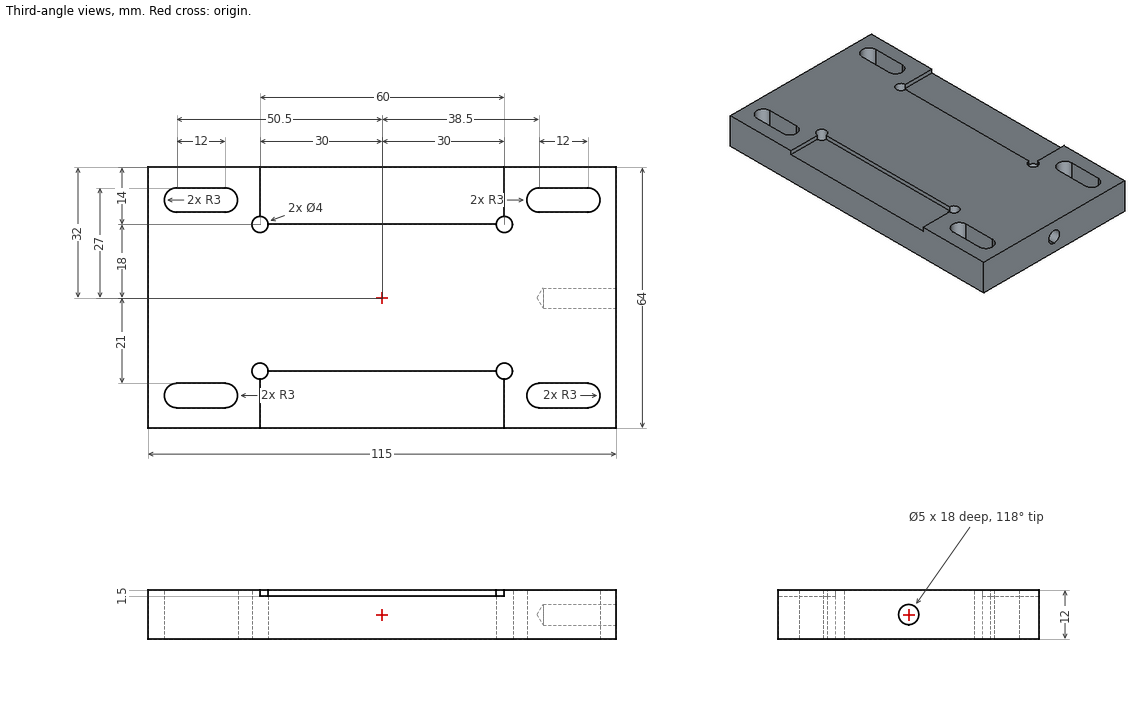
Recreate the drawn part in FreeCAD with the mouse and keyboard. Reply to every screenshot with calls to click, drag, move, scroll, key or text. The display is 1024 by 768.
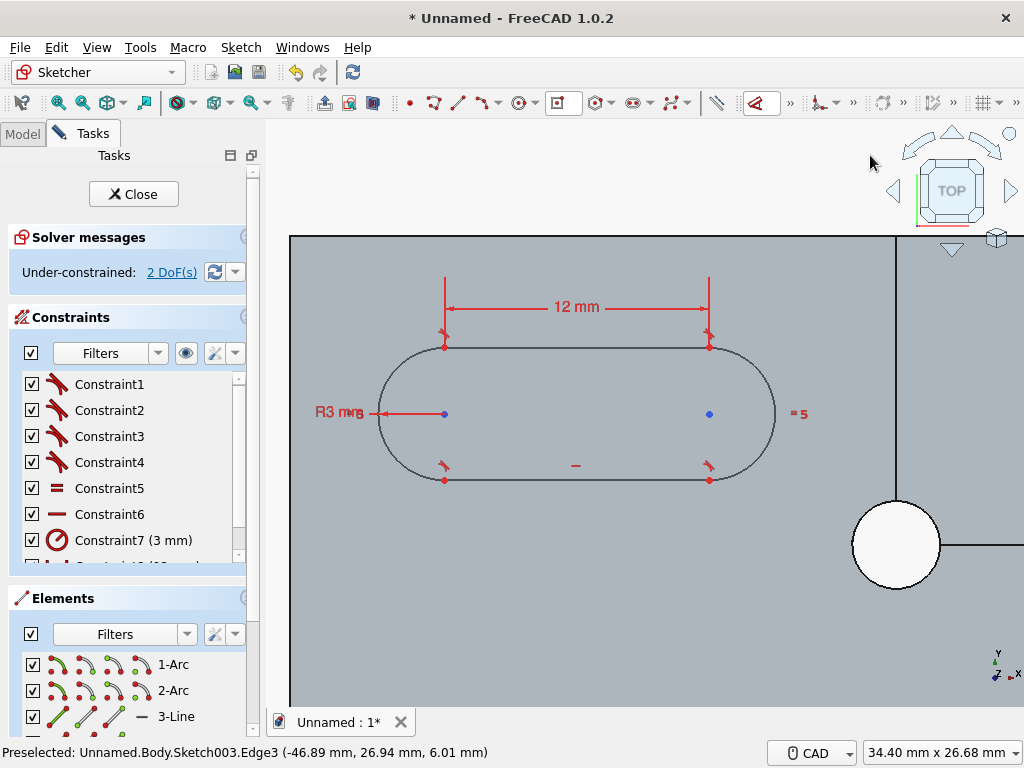
click(445, 348)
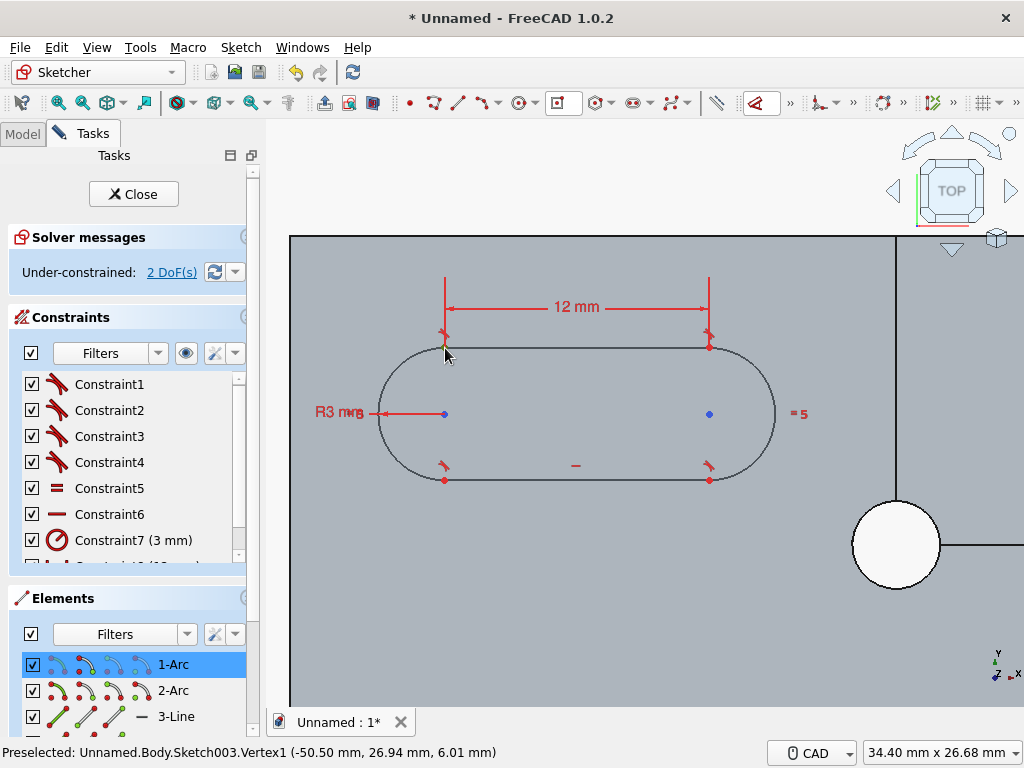
key(i)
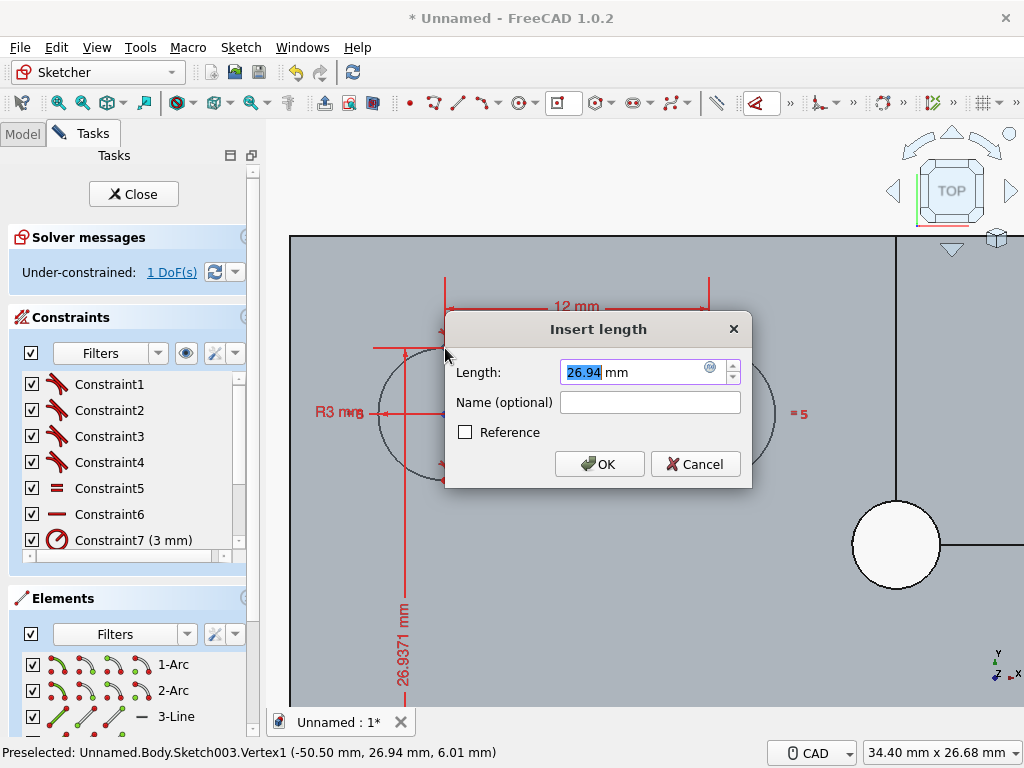
text(27)
key(Return)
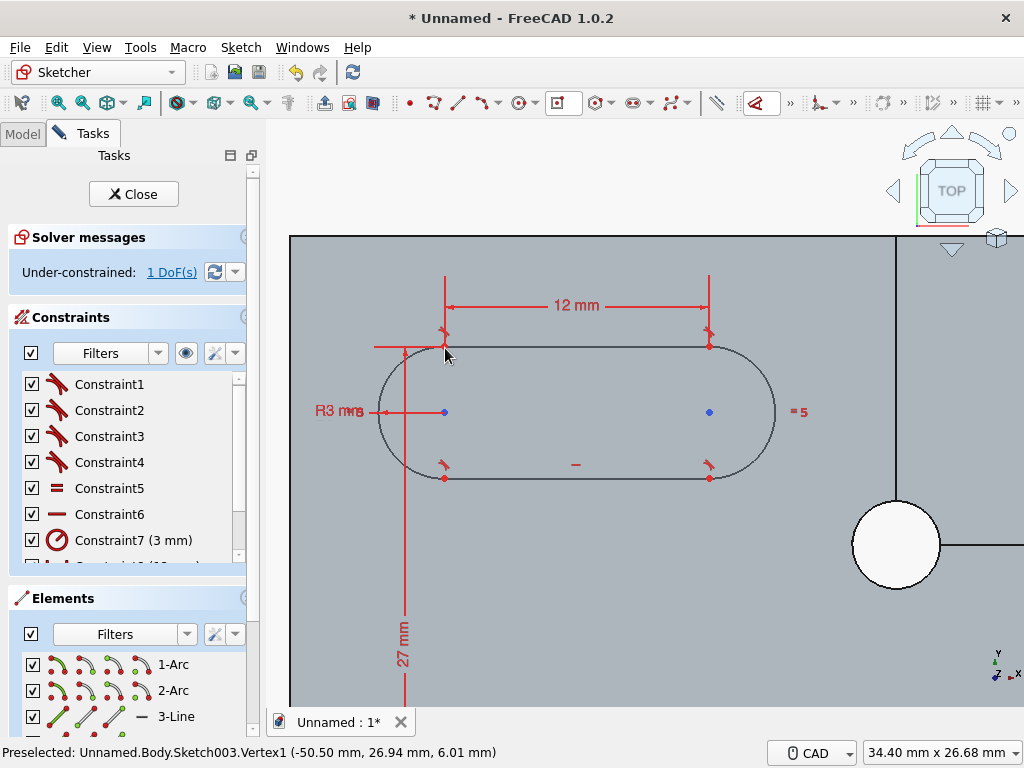
click(445, 347)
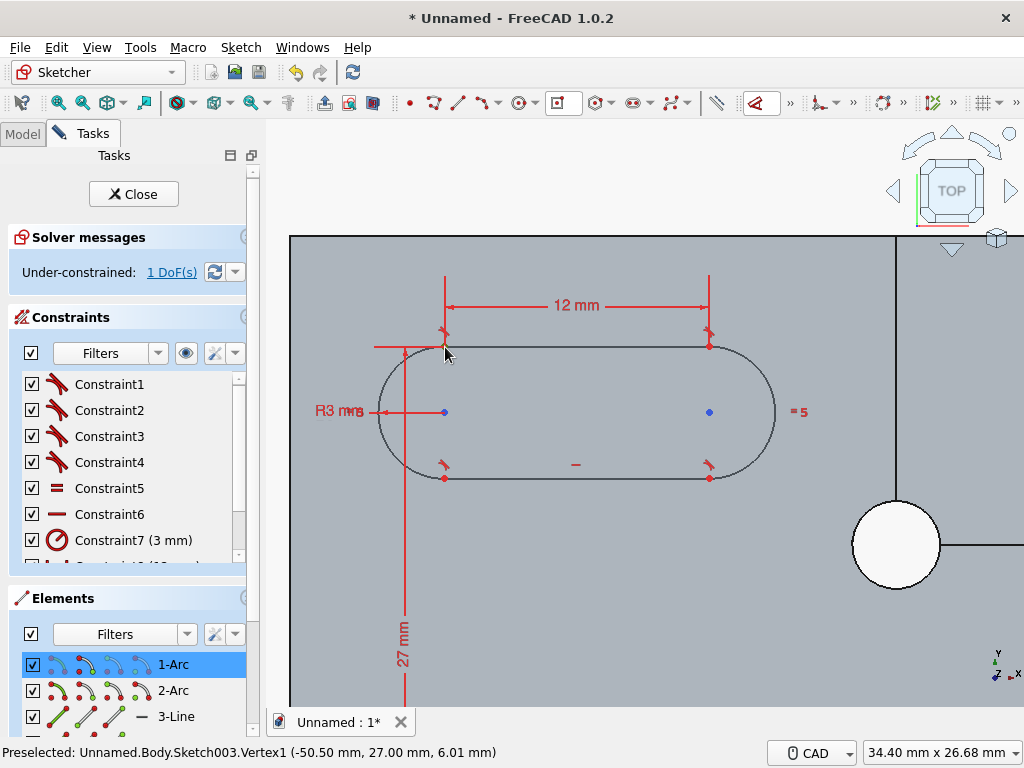
key(l)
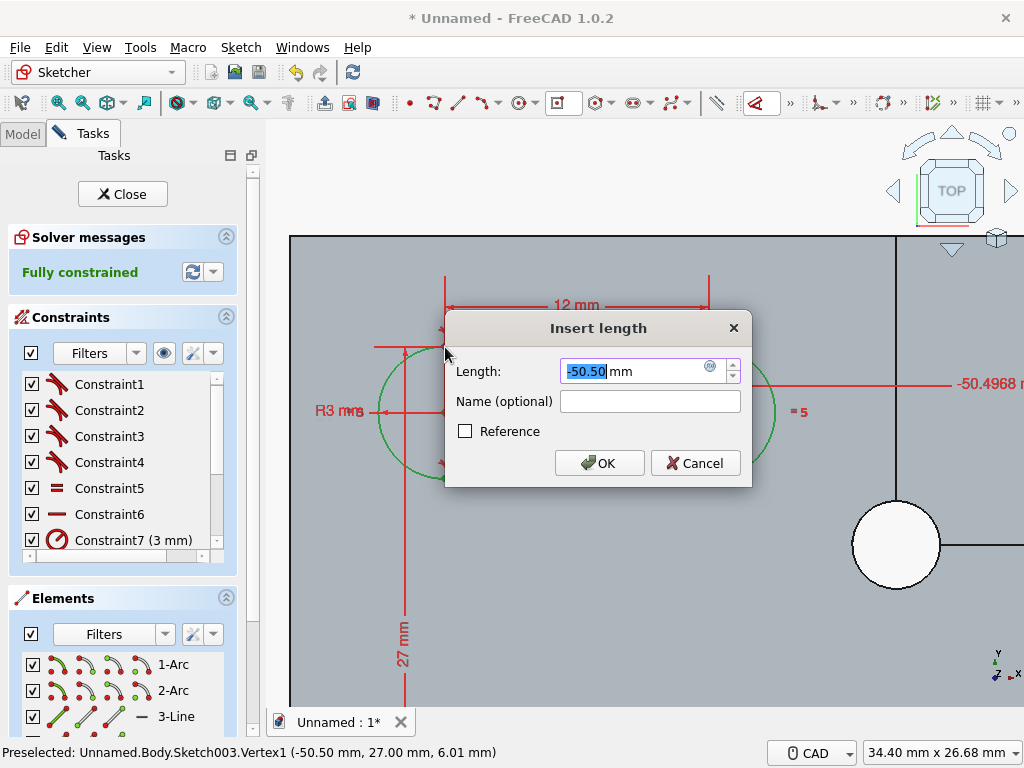
text(-50.5)
key(Return)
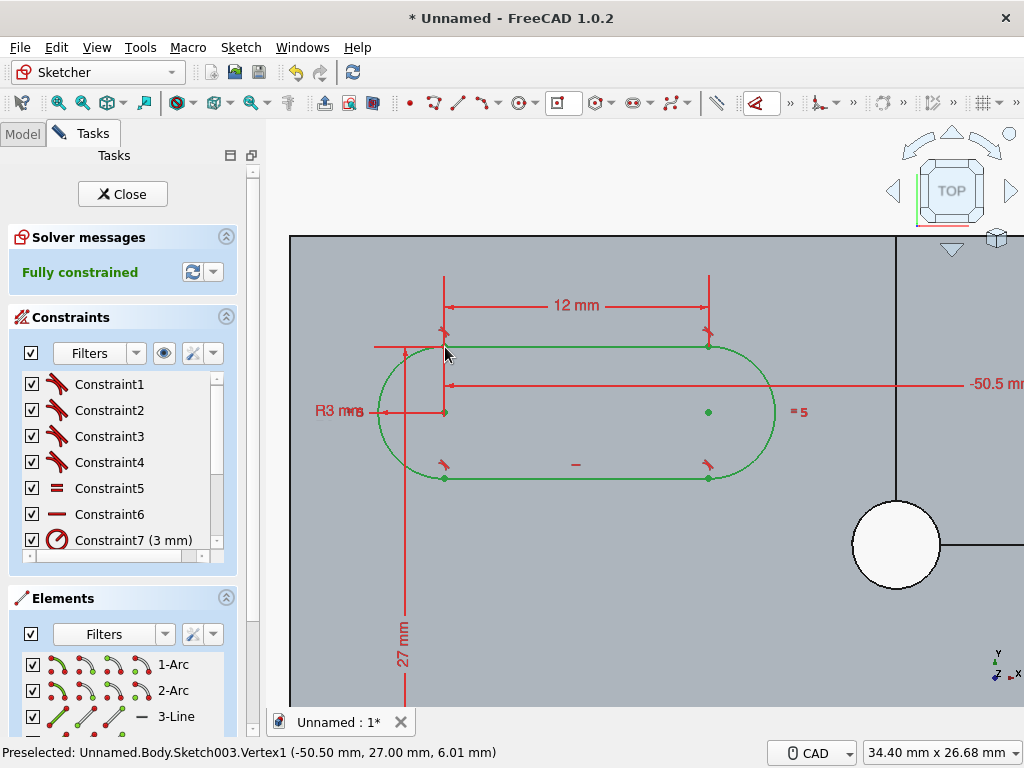
click(123, 194)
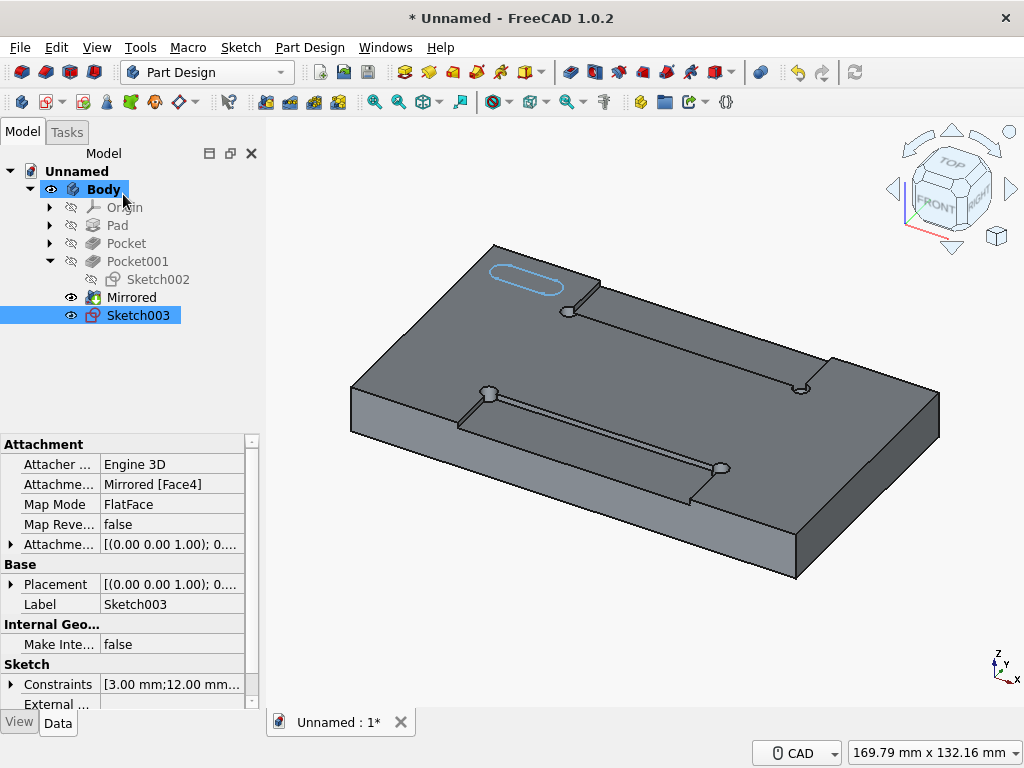
click(572, 72)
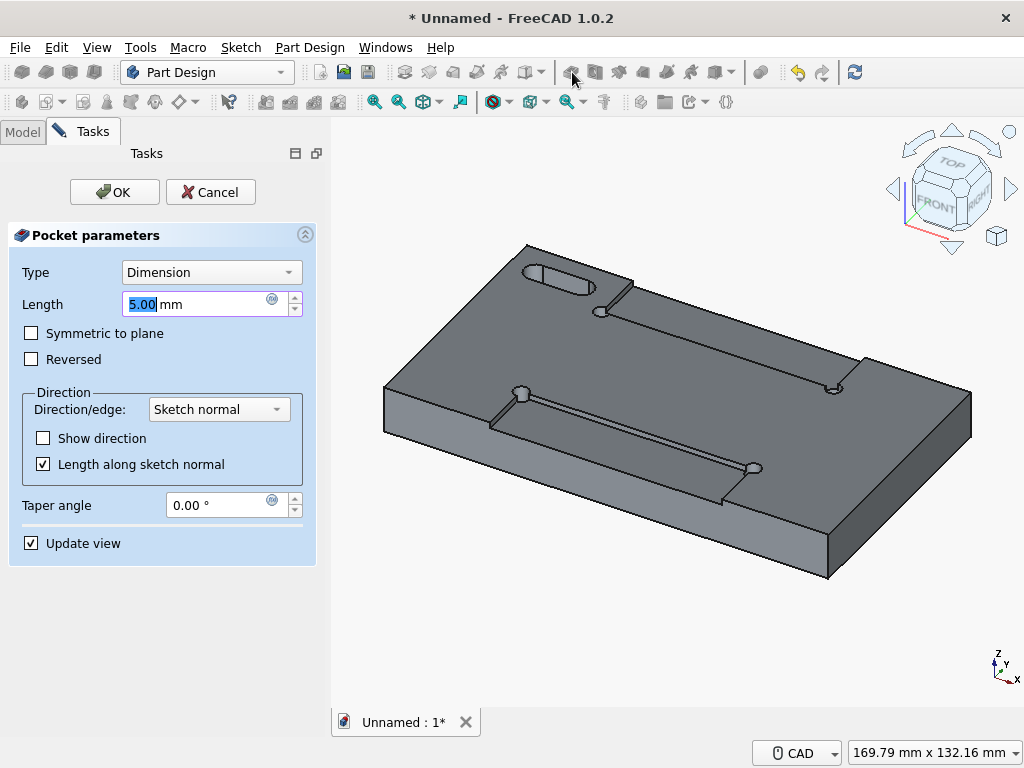
click(212, 272)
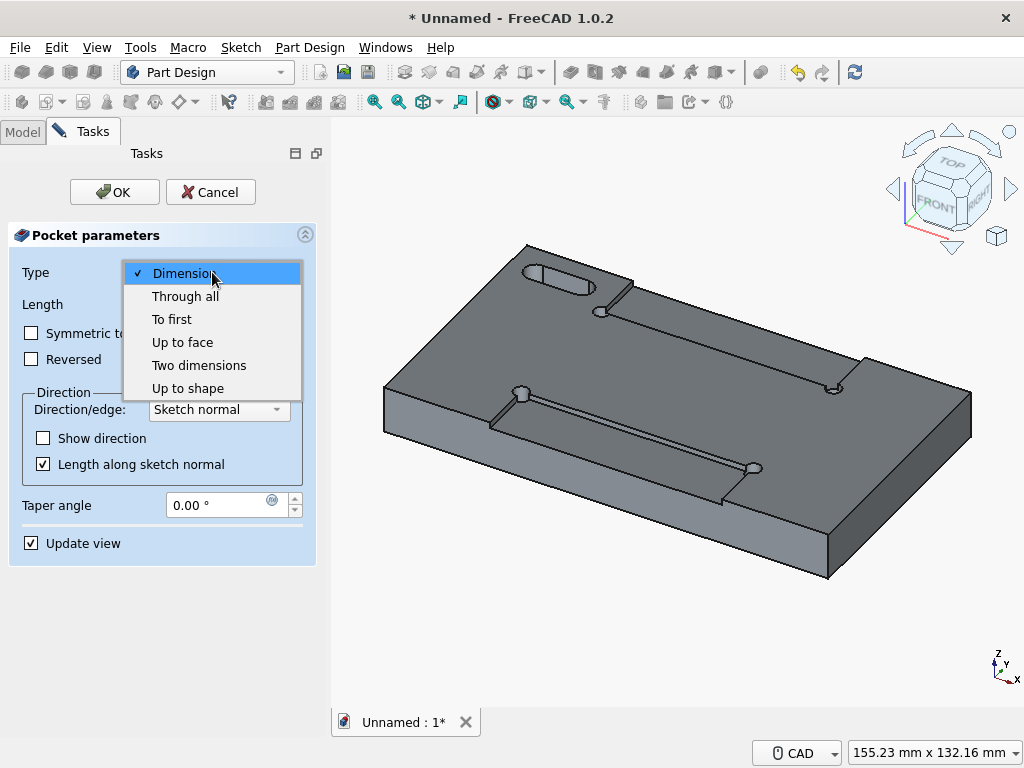
click(212, 320)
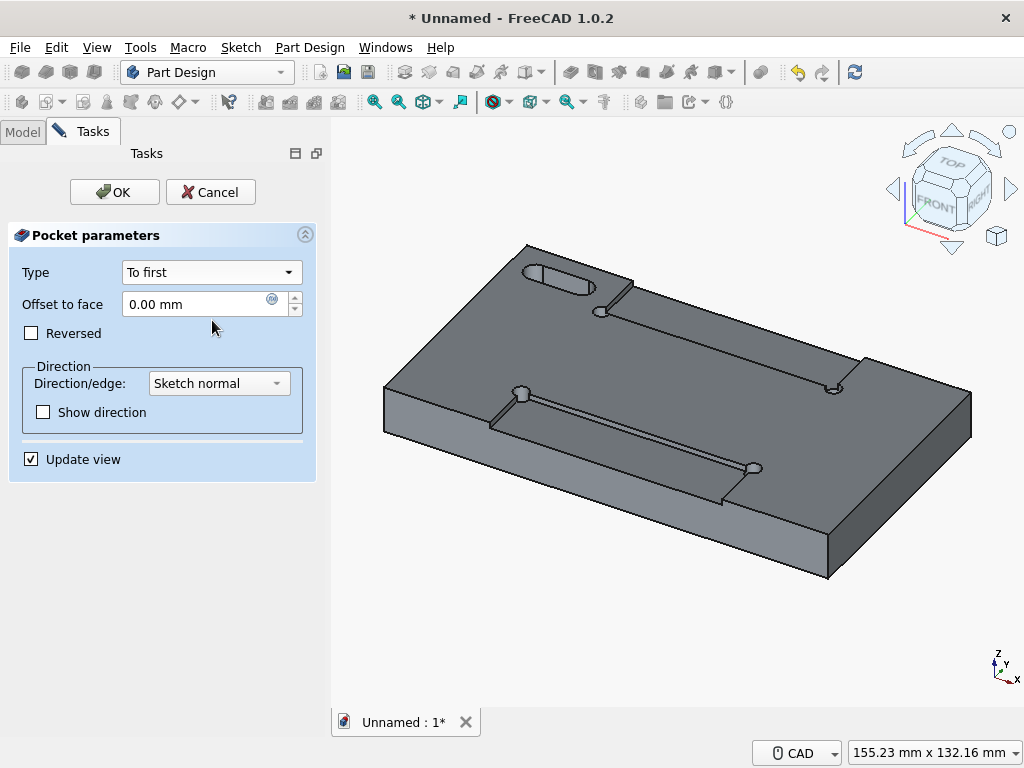
click(115, 192)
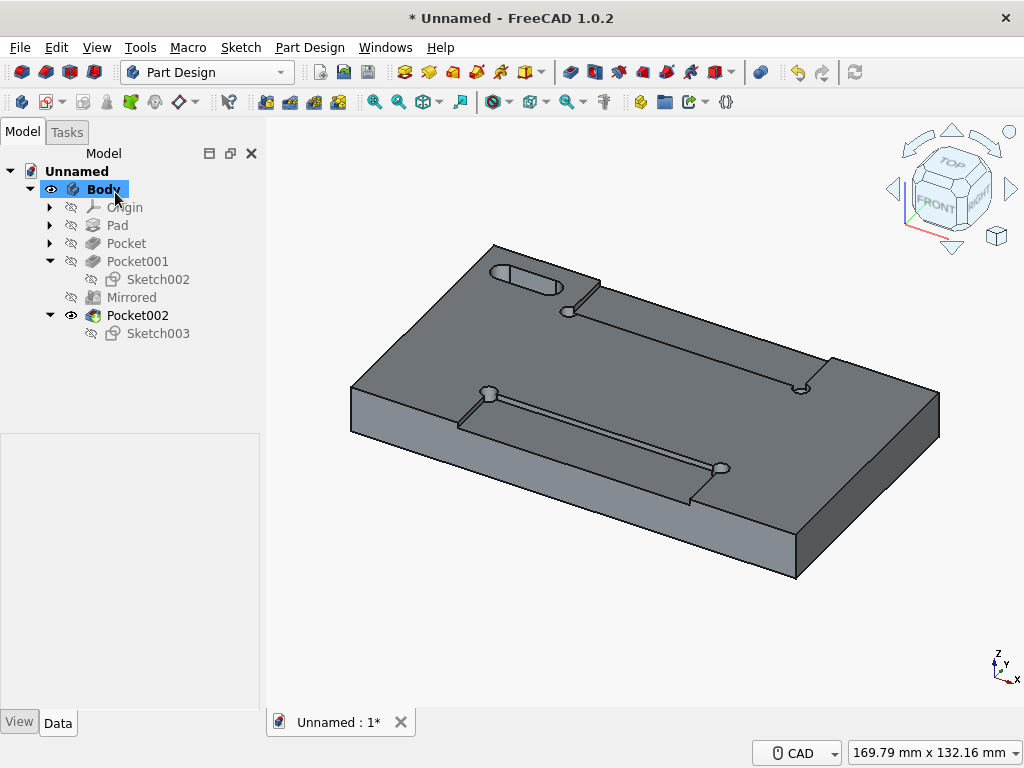
click(709, 410)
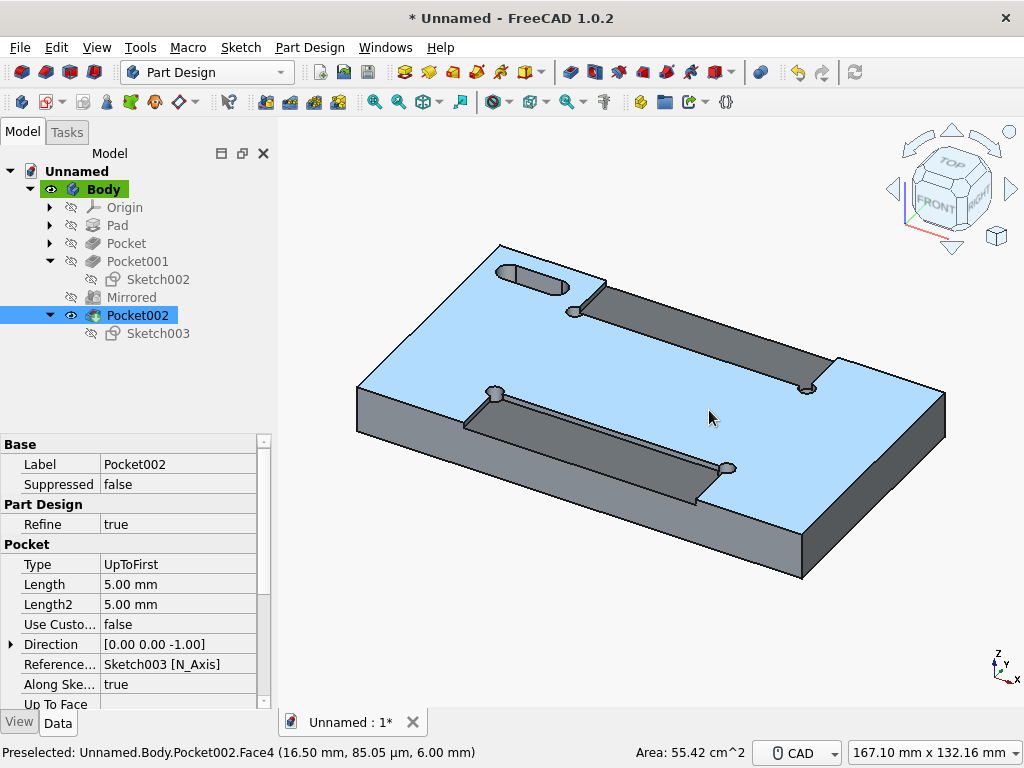
click(46, 102)